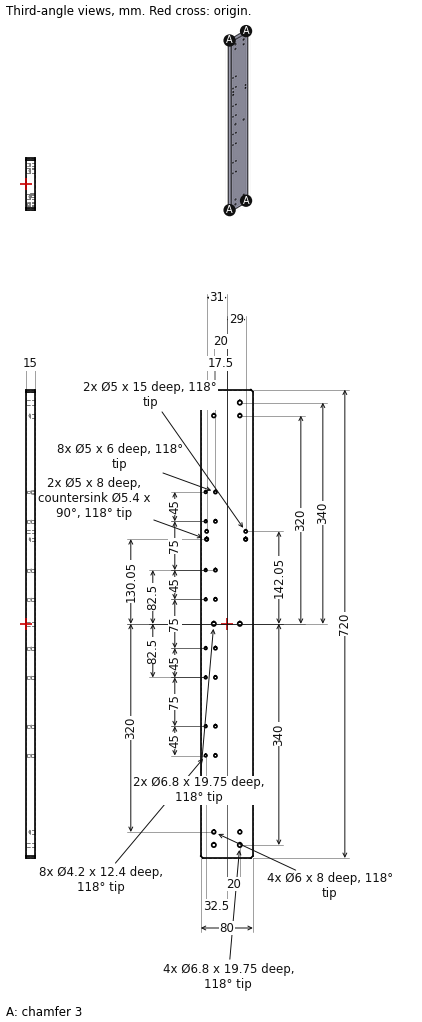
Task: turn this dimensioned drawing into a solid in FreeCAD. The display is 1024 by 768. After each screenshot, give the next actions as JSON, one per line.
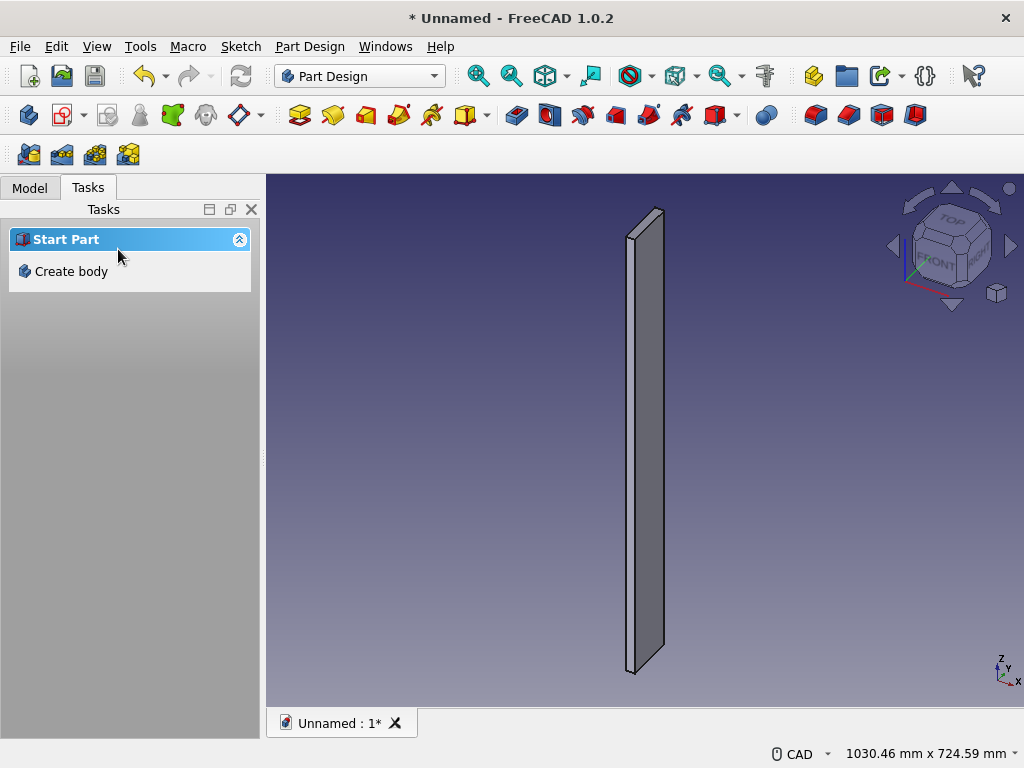
{"action": "left_click", "coordinate": [650, 441]}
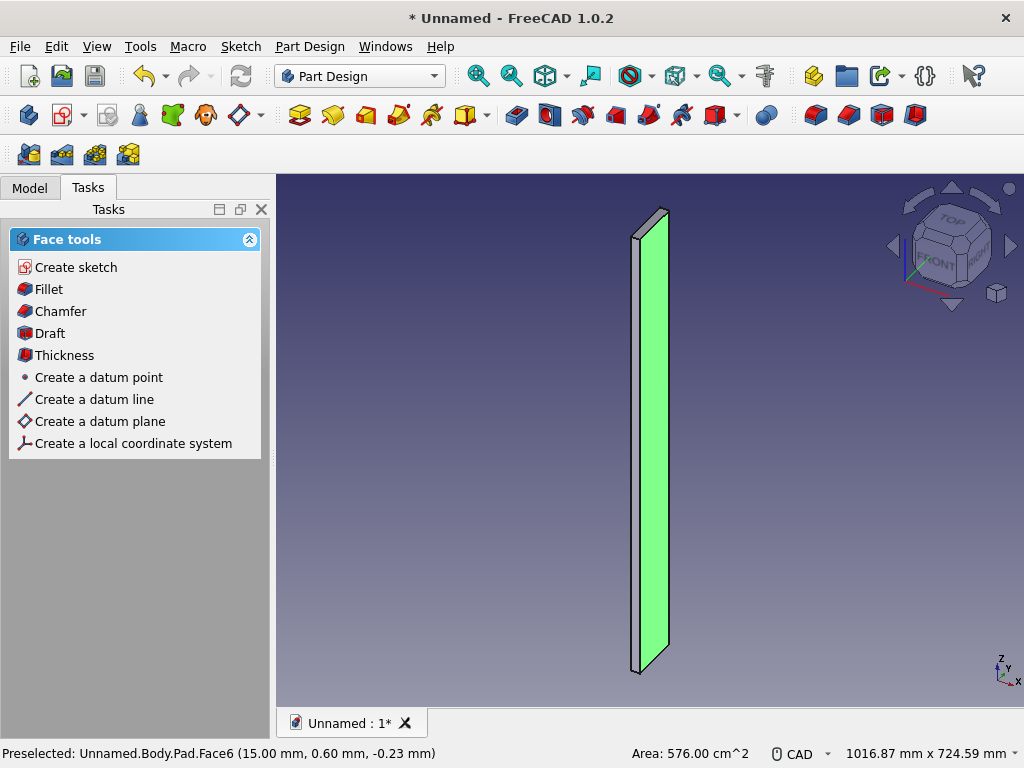
{"action": "left_click", "coordinate": [62, 116]}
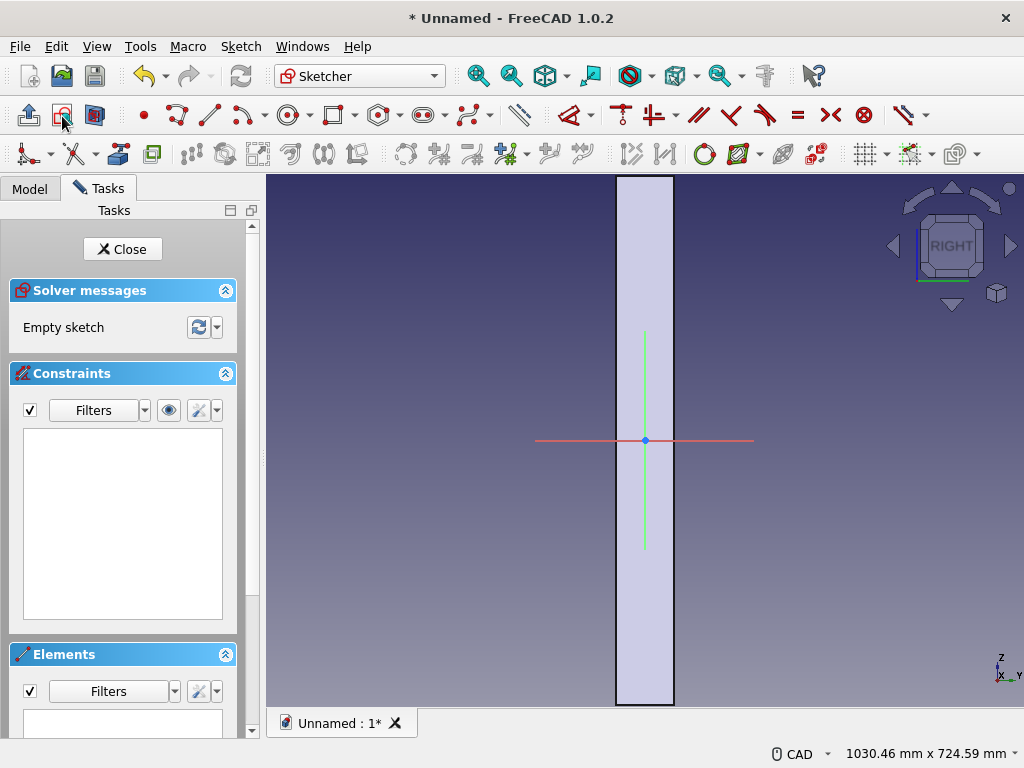
{"action": "left_click", "coordinate": [288, 116]}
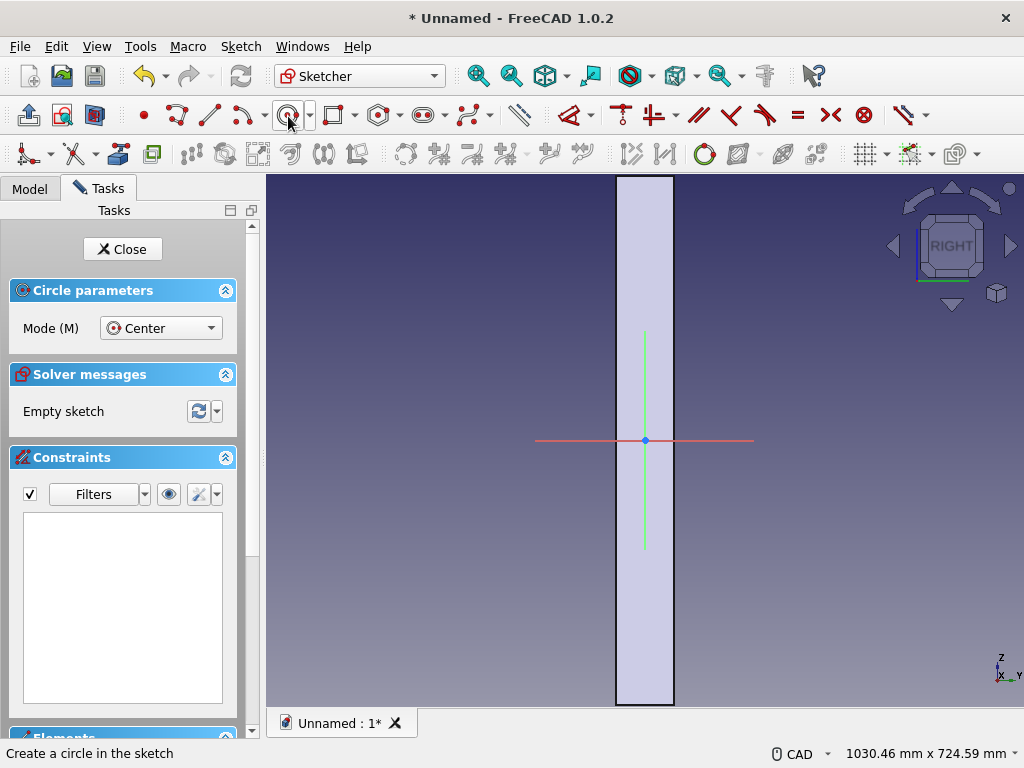
{"action": "scroll", "coordinate": [621, 589], "scroll_direction": "up", "scroll_amount": 14}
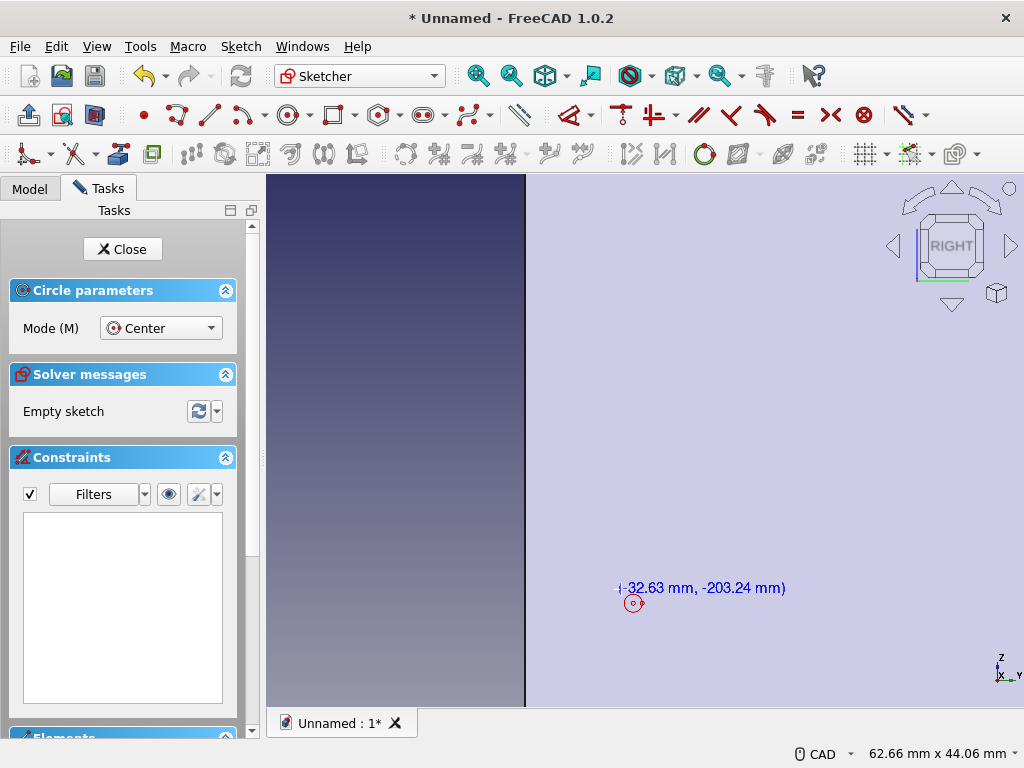
{"action": "scroll", "coordinate": [559, 625], "scroll_direction": "down", "scroll_amount": 13}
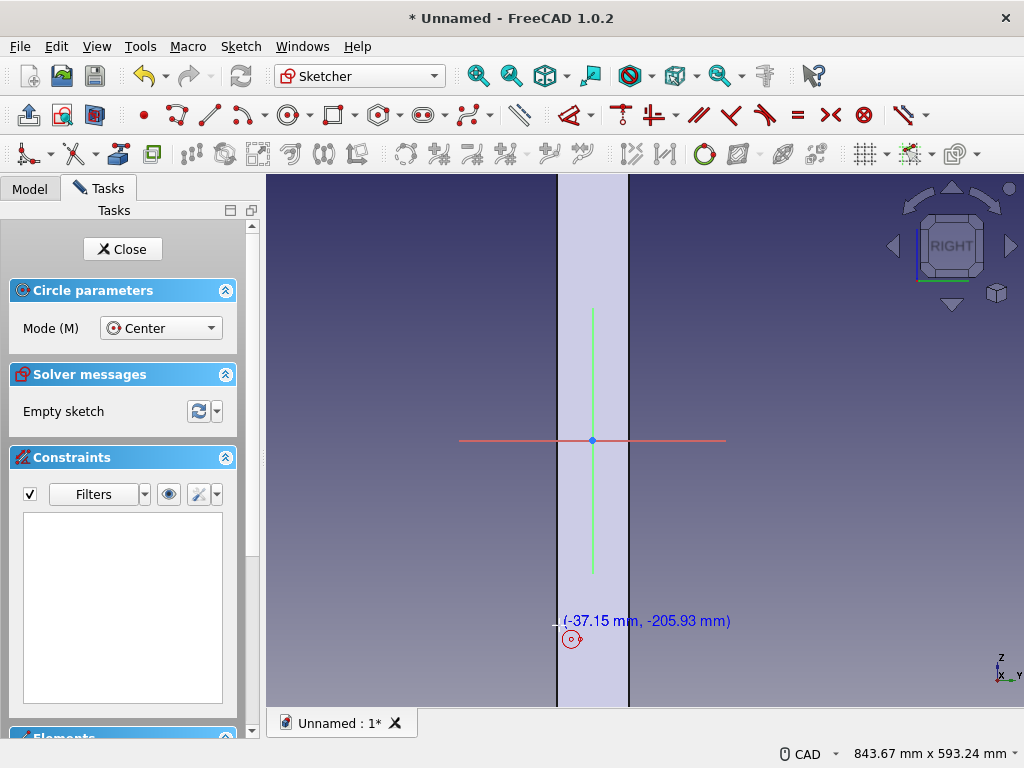
{"action": "left_click", "coordinate": [564, 623]}
{"action": "mouse_move", "coordinate": [565, 621]}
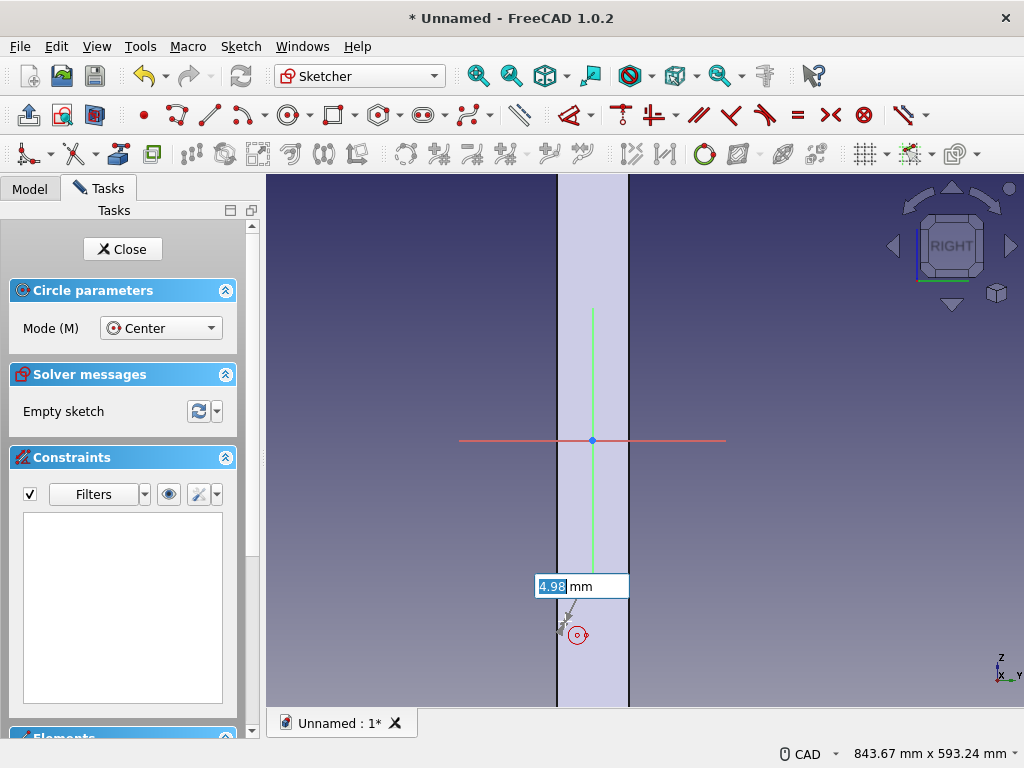
{"action": "type", "text": "4.2"}
{"action": "key", "text": "Return"}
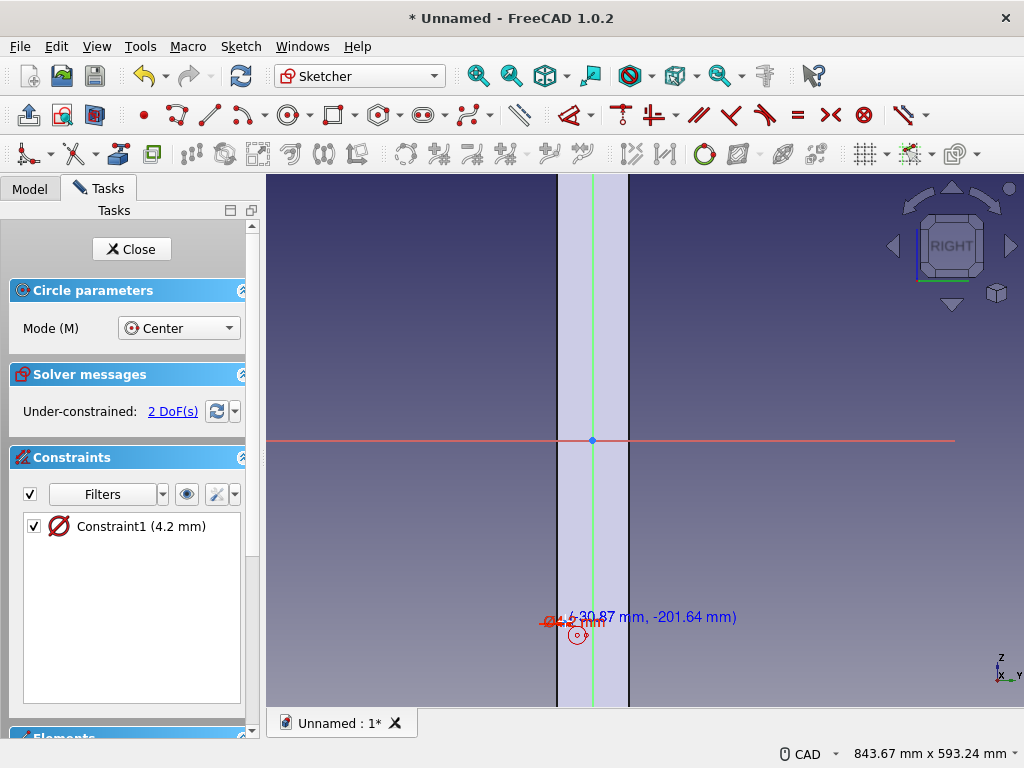
{"action": "scroll", "coordinate": [564, 582], "scroll_direction": "up", "scroll_amount": 13}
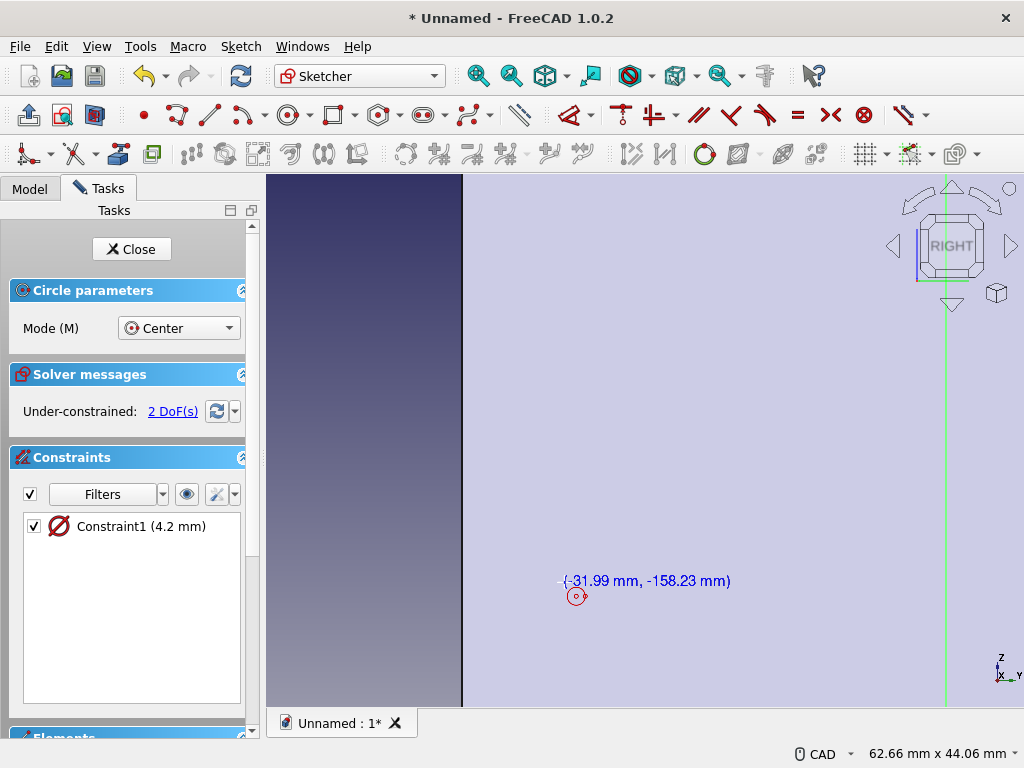
{"action": "scroll", "coordinate": [564, 582], "scroll_direction": "down", "scroll_amount": 13}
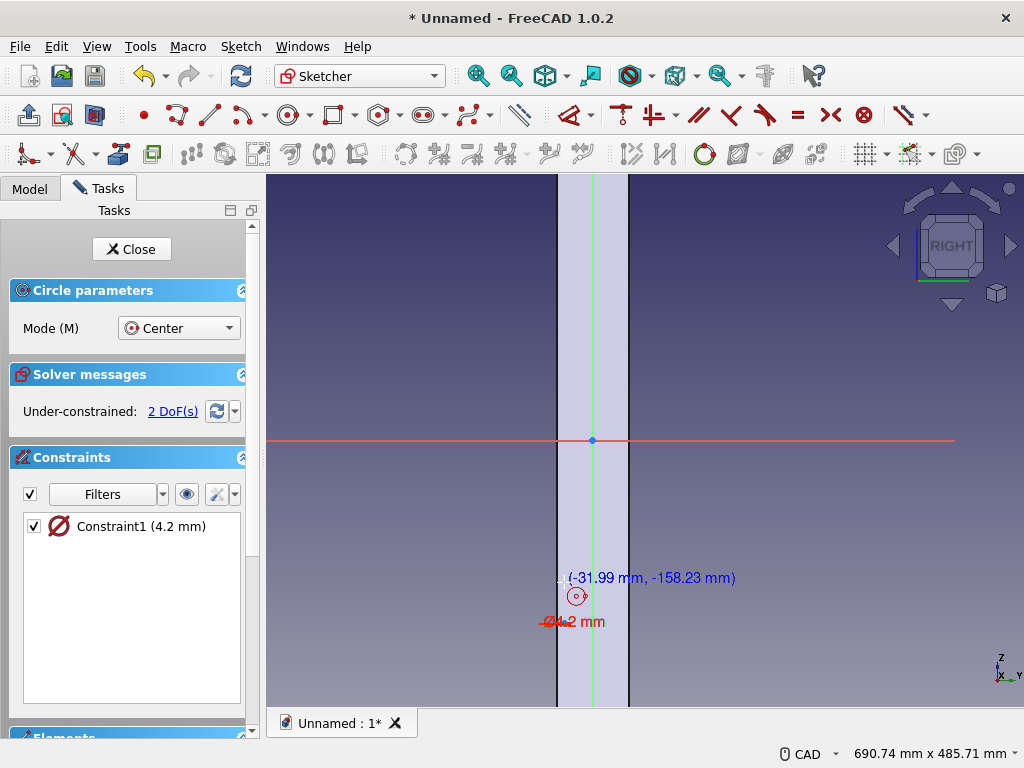
{"action": "left_click", "coordinate": [564, 582]}
{"action": "mouse_move", "coordinate": [565, 581]}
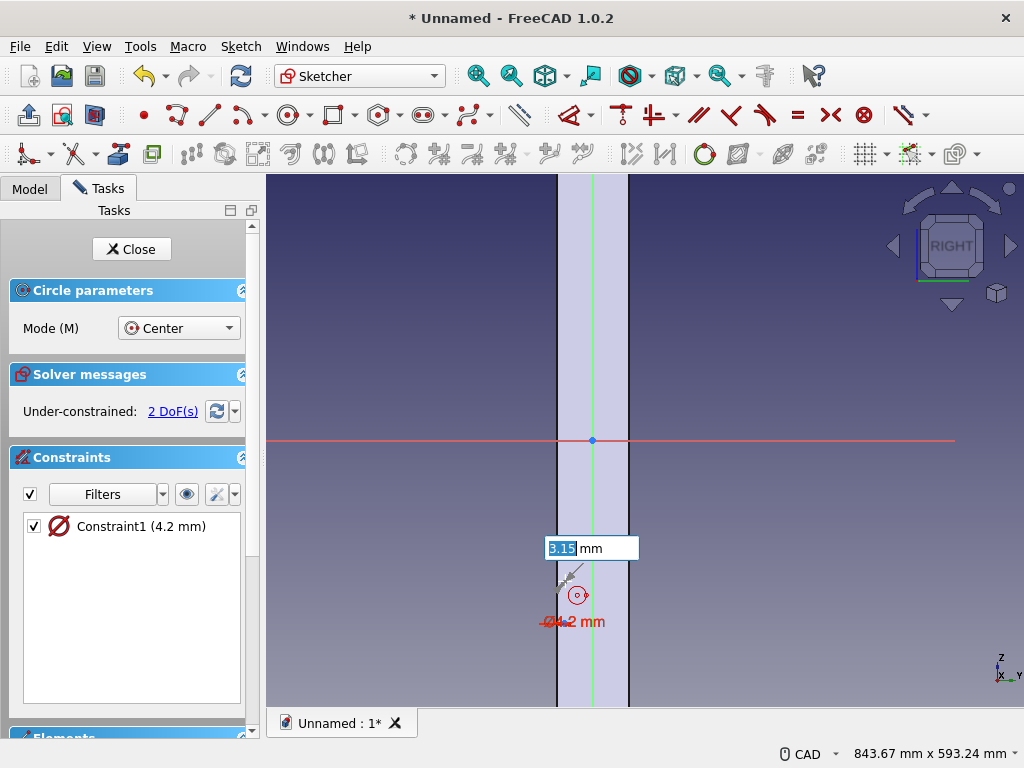
{"action": "type", "text": "4.2"}
{"action": "key", "text": "Return"}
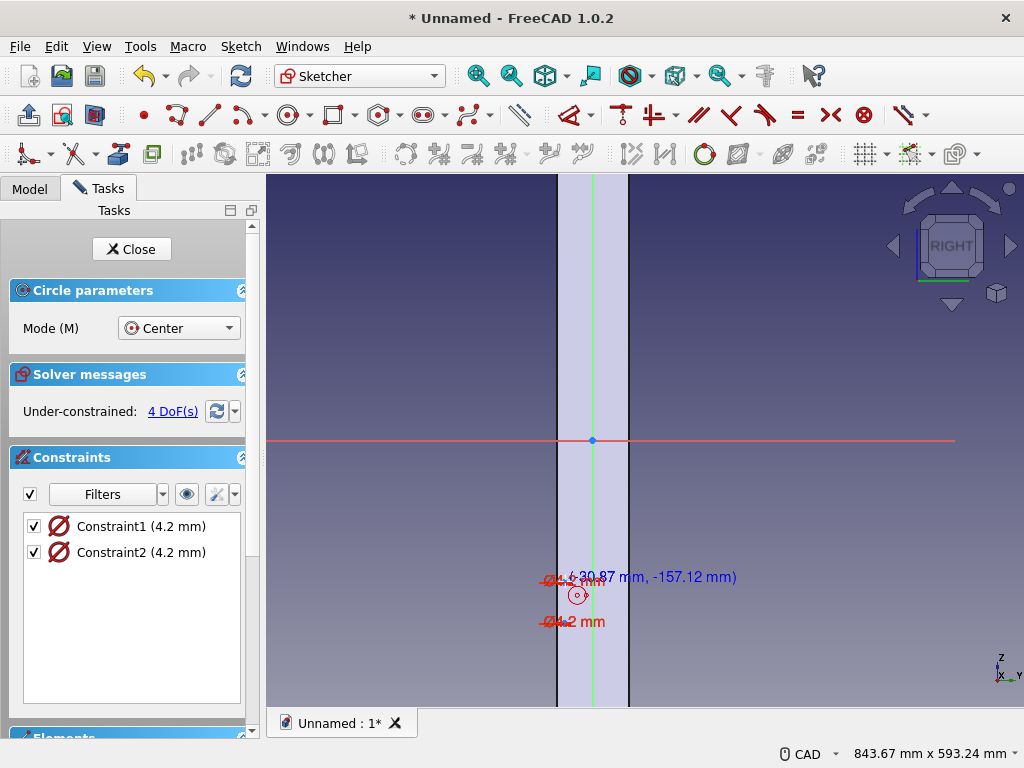
{"action": "scroll", "coordinate": [564, 515], "scroll_direction": "up", "scroll_amount": 13}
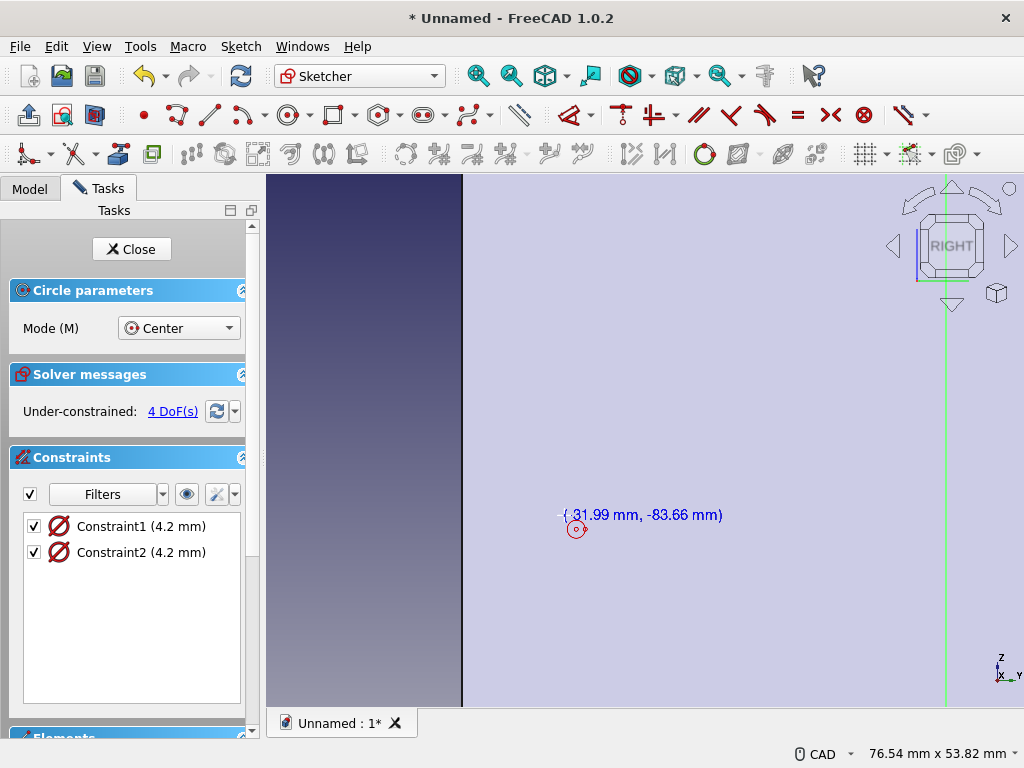
{"action": "scroll", "coordinate": [564, 515], "scroll_direction": "down", "scroll_amount": 13}